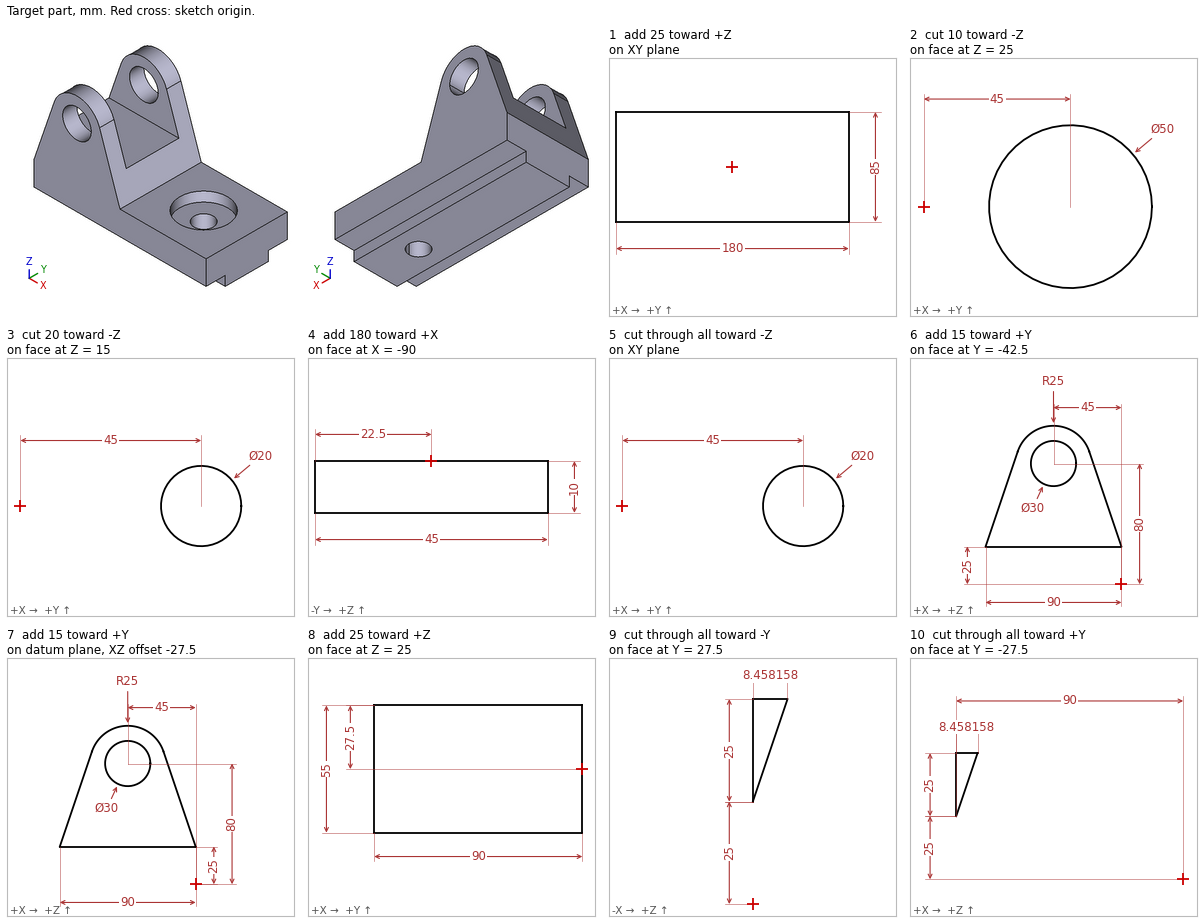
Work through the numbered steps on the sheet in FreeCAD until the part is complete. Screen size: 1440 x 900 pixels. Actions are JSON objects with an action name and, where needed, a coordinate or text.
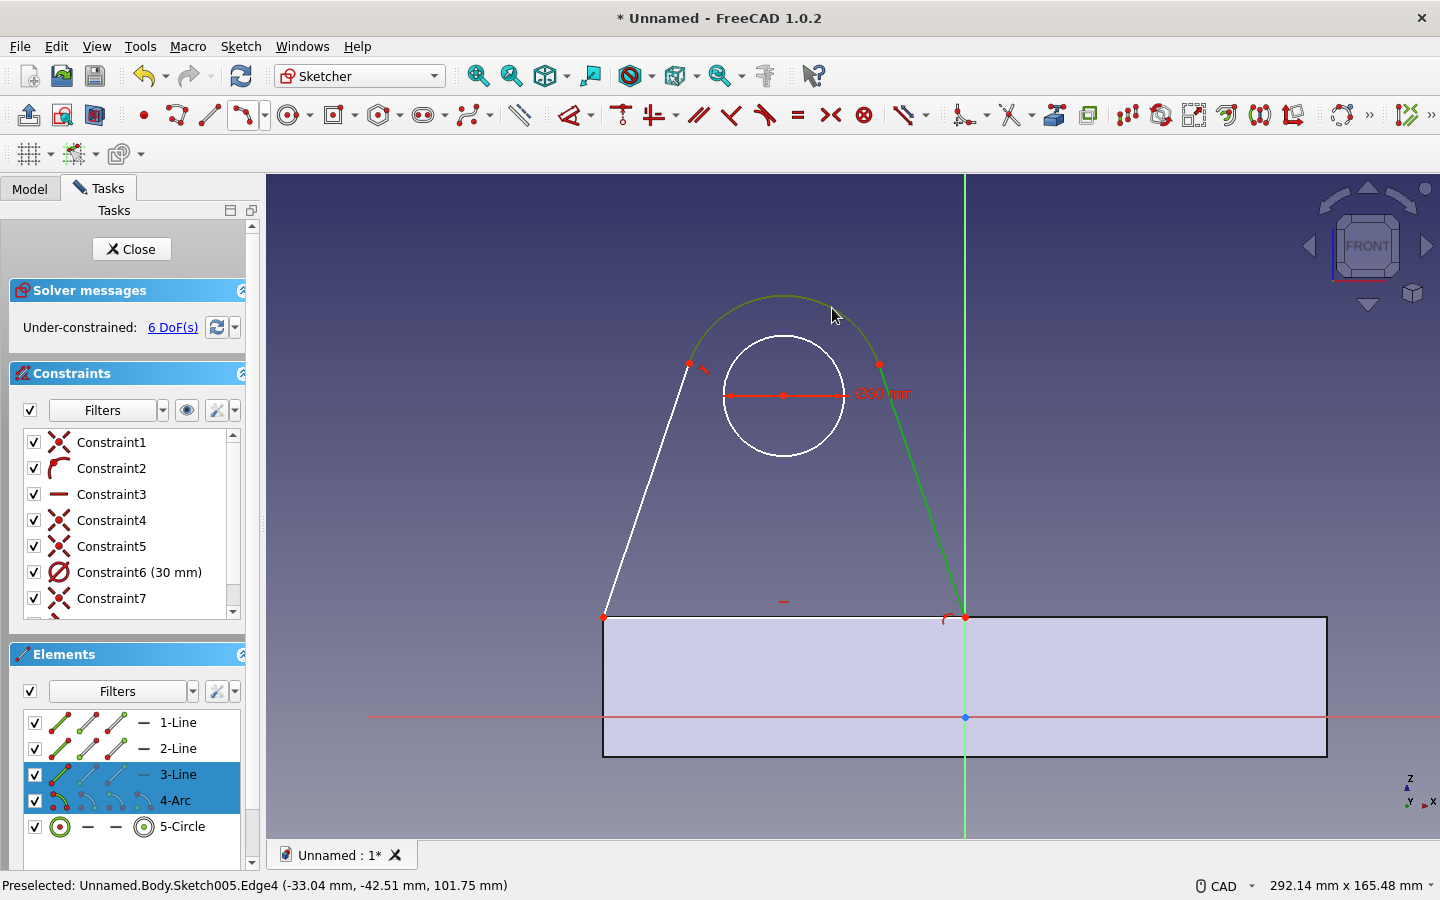
{"action": "left_click", "coordinate": [765, 116]}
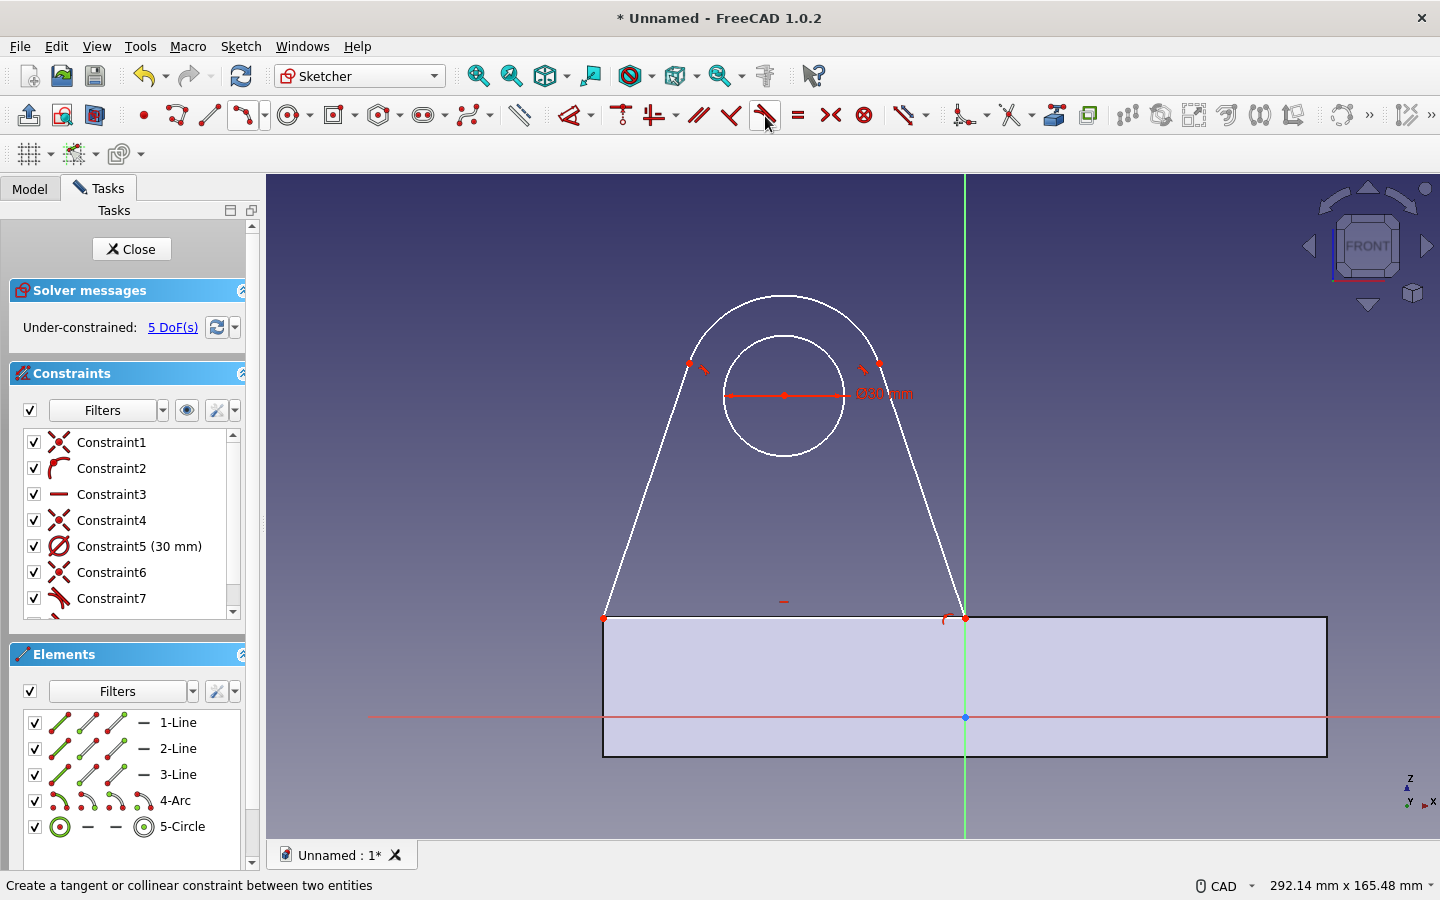
{"action": "left_click", "coordinate": [568, 116]}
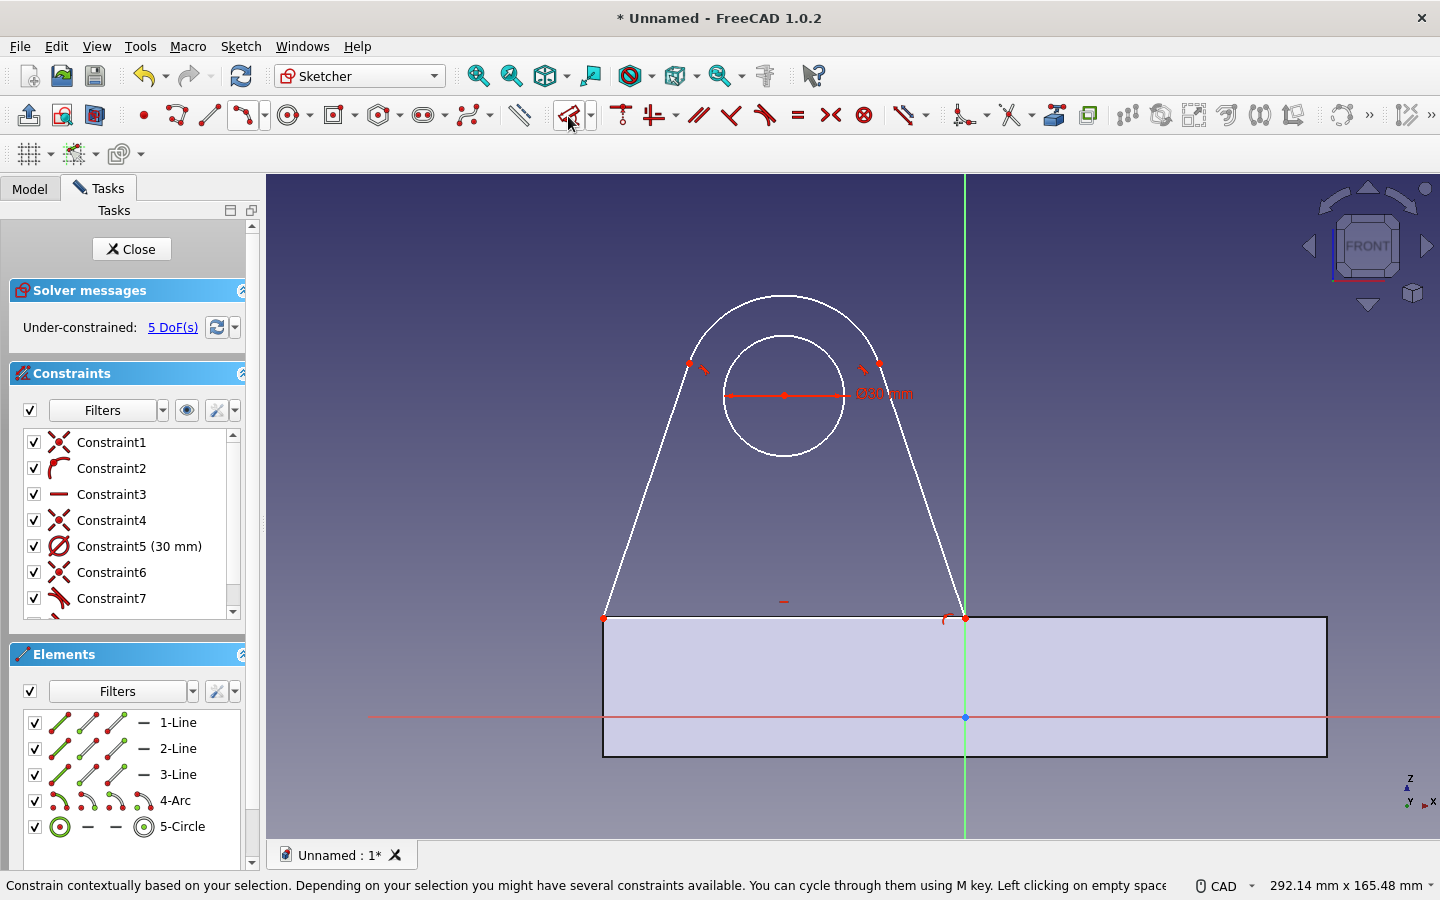
{"action": "left_click", "coordinate": [832, 308]}
{"action": "left_click", "coordinate": [847, 280]}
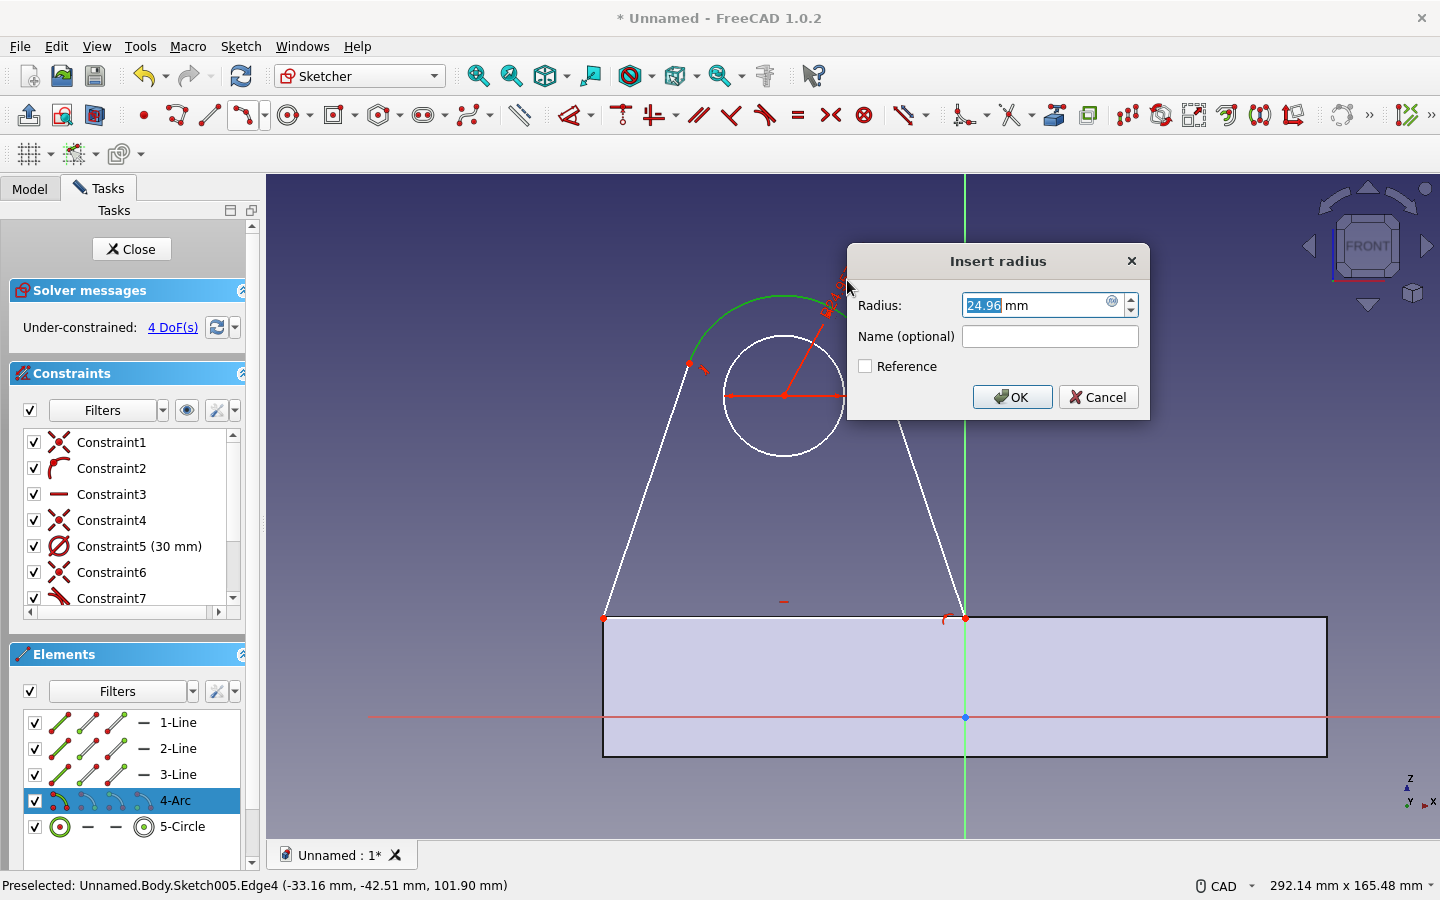
{"action": "type", "text": "25"}
{"action": "key", "text": "Return"}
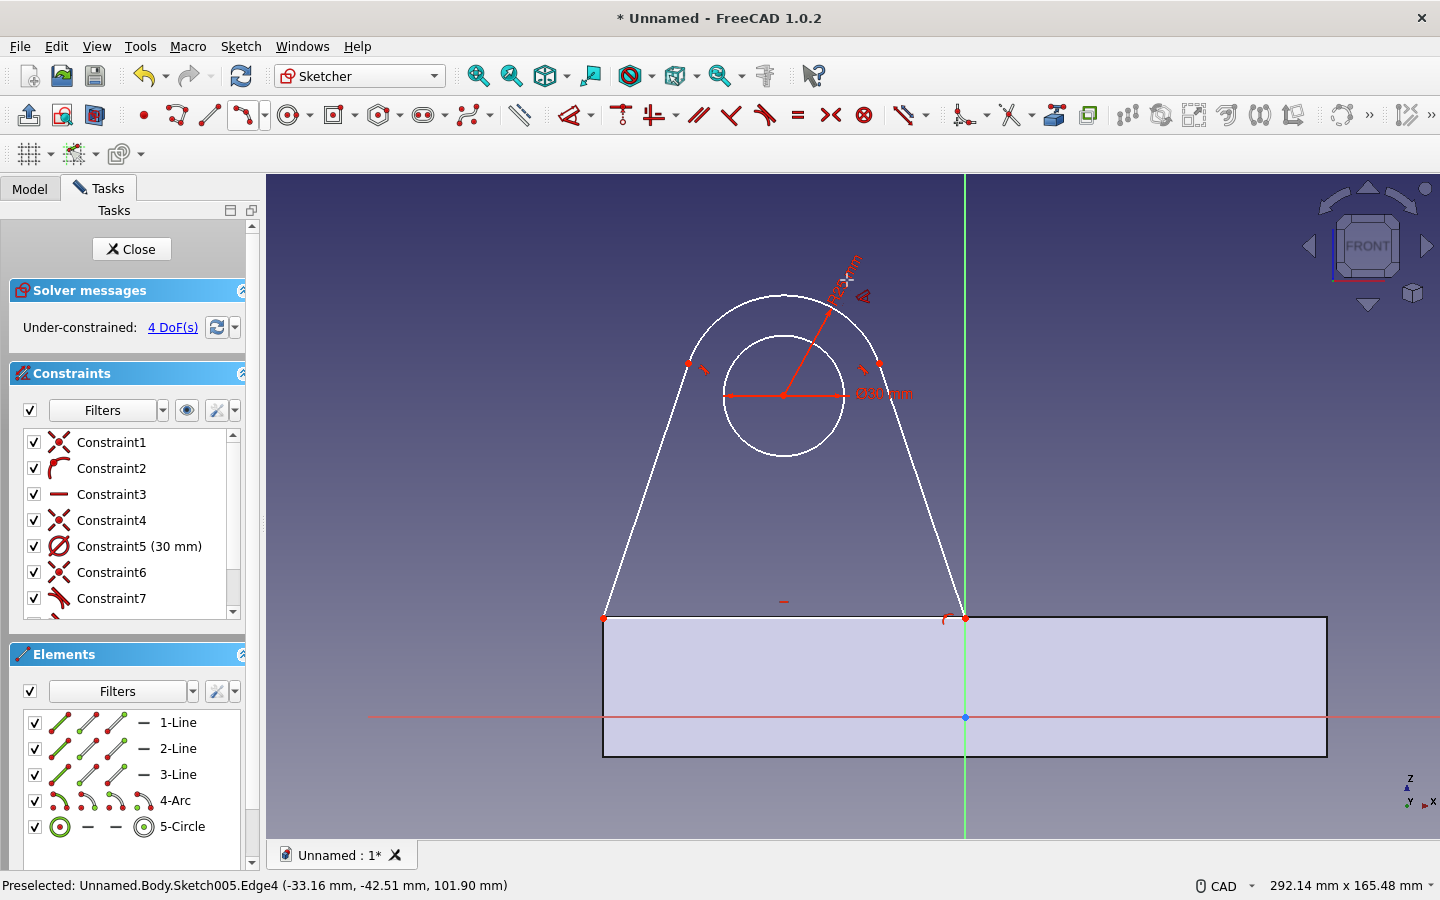
{"action": "left_click", "coordinate": [712, 618]}
{"action": "left_click", "coordinate": [784, 652]}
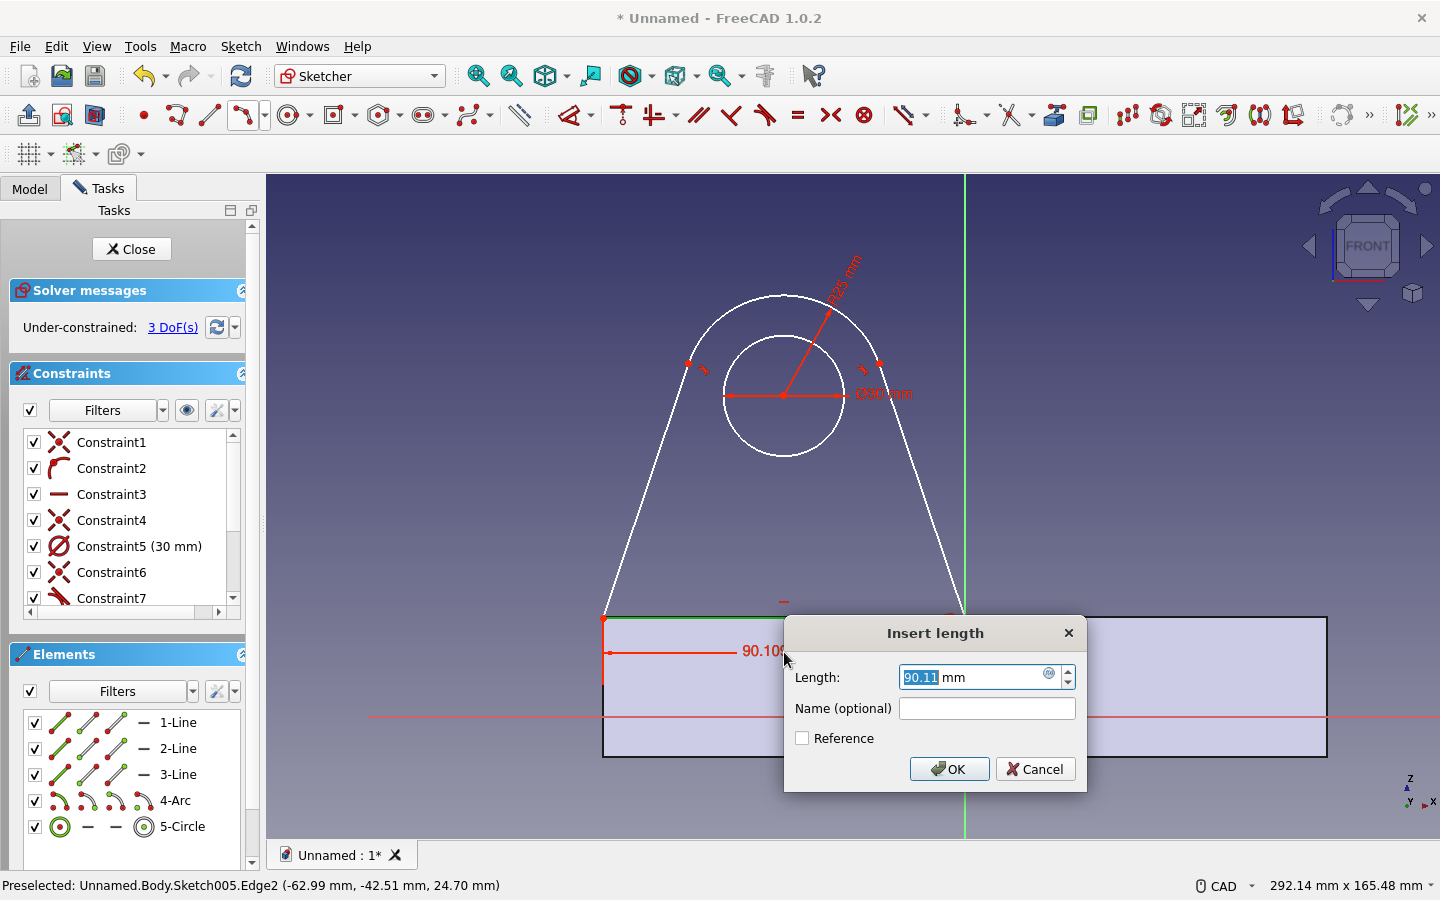
{"action": "type", "text": "90"}
{"action": "key", "text": "Return"}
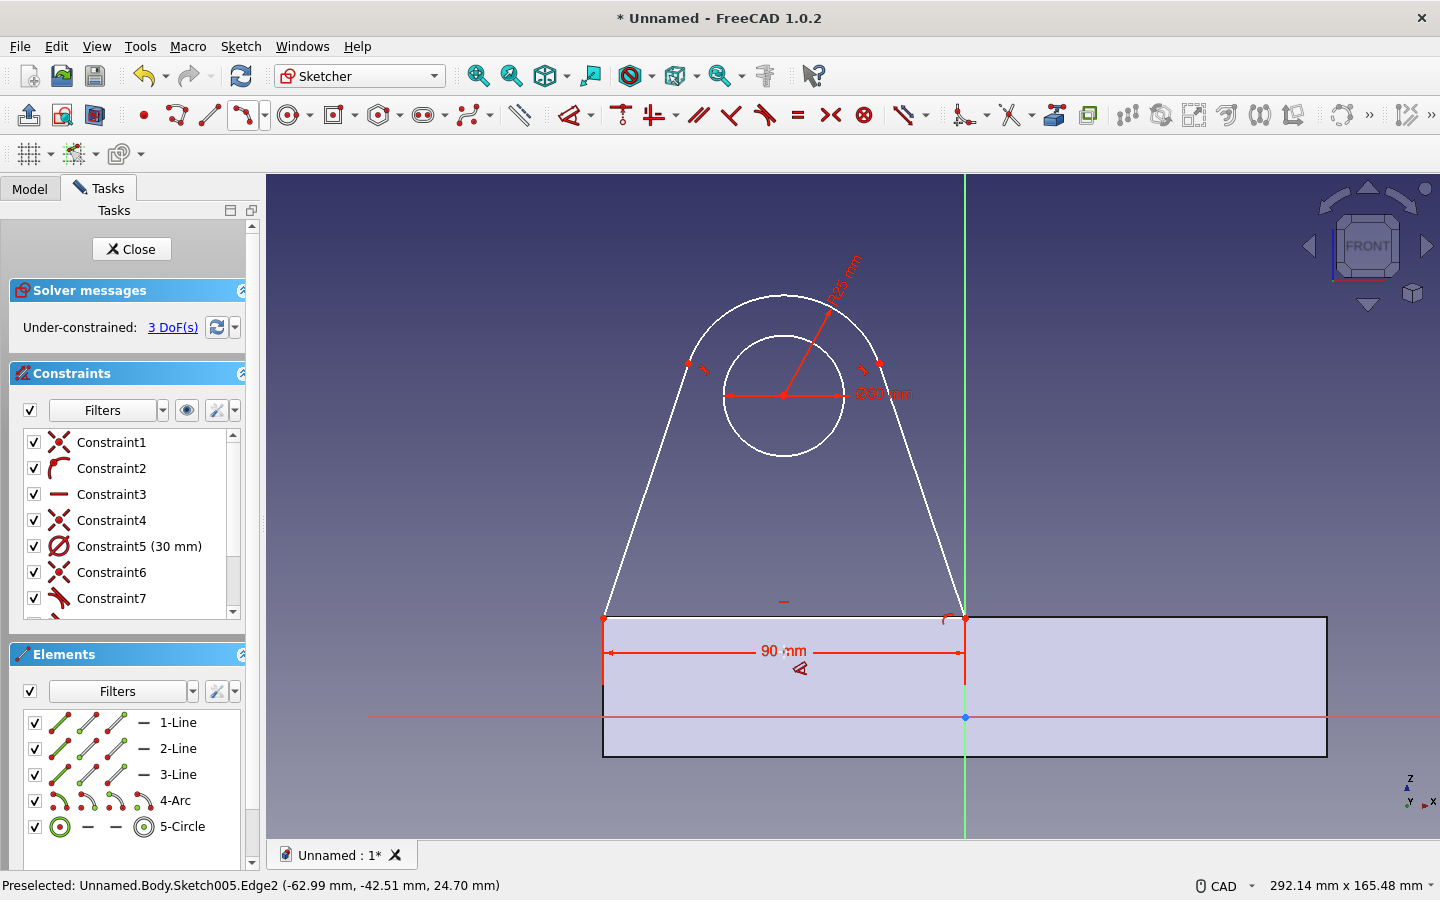
{"action": "left_click", "coordinate": [784, 396]}
{"action": "left_click", "coordinate": [874, 751]}